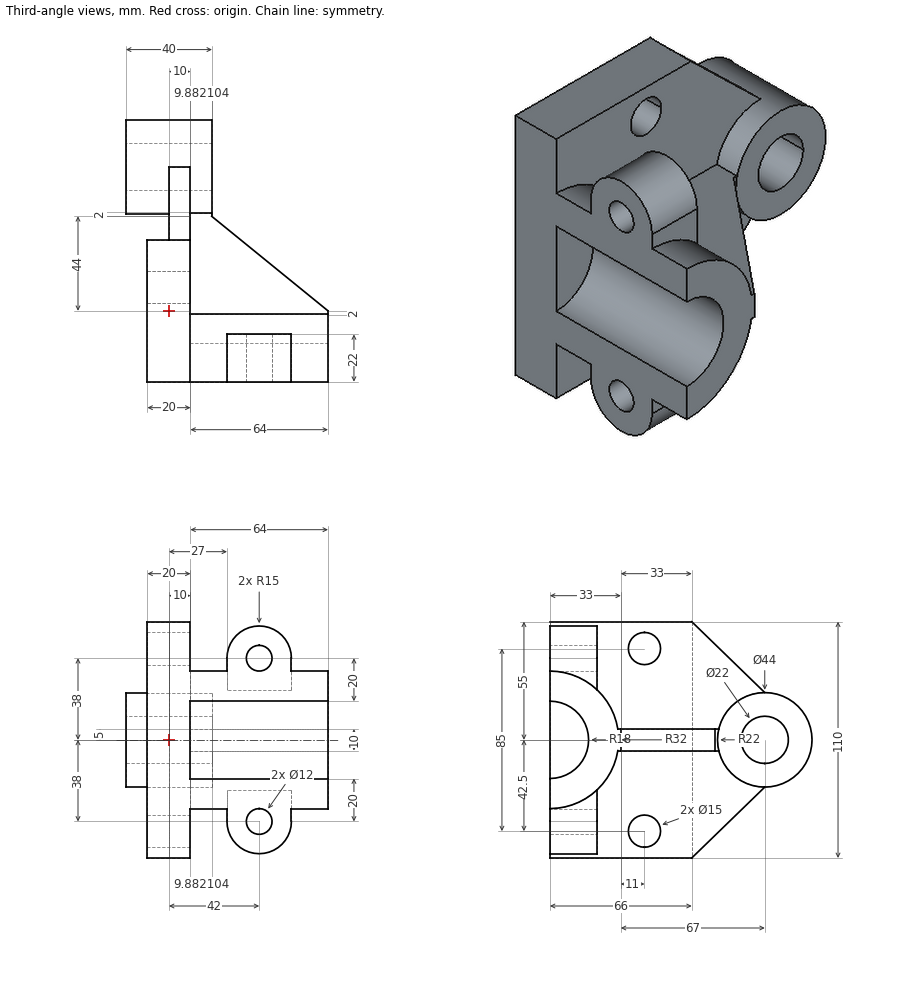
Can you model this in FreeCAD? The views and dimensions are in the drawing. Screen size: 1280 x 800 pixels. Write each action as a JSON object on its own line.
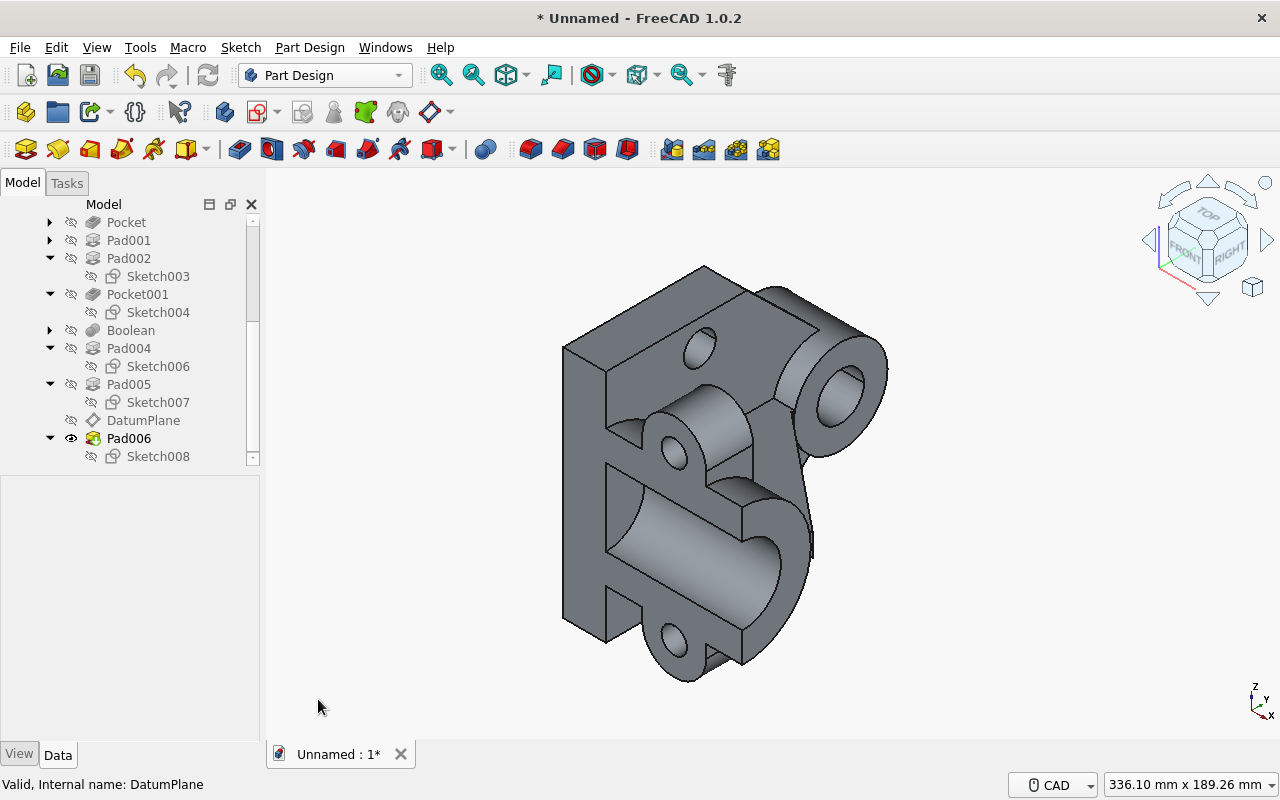
{"action": "left_click", "coordinate": [258, 112]}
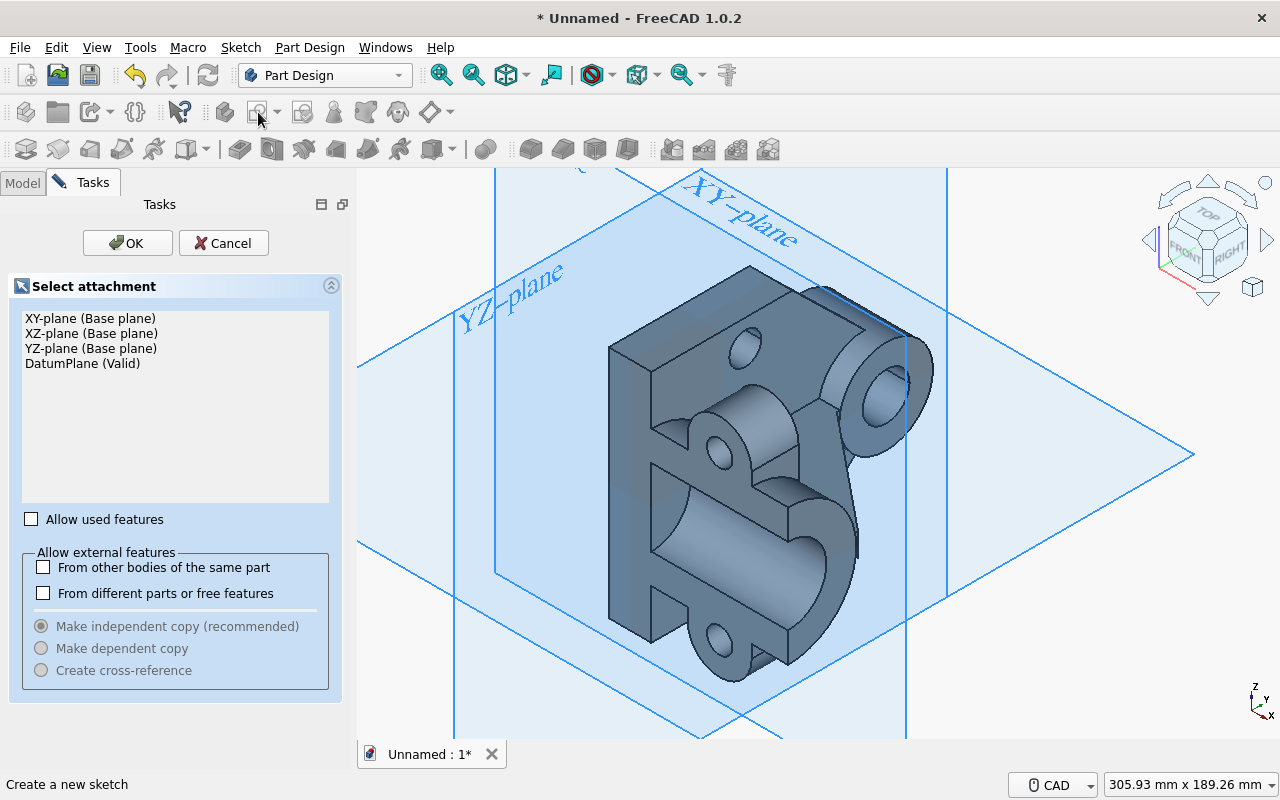
{"action": "left_click", "coordinate": [82, 334]}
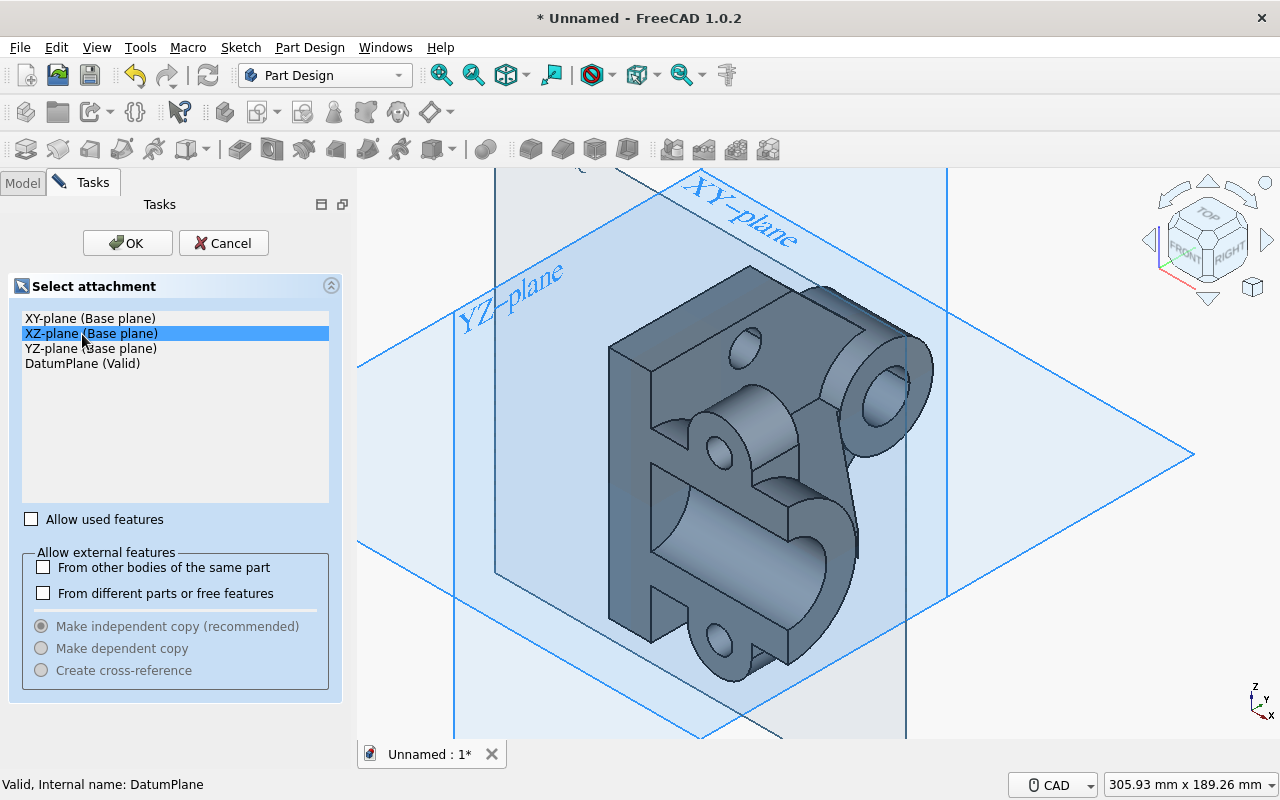
{"action": "left_click", "coordinate": [128, 243]}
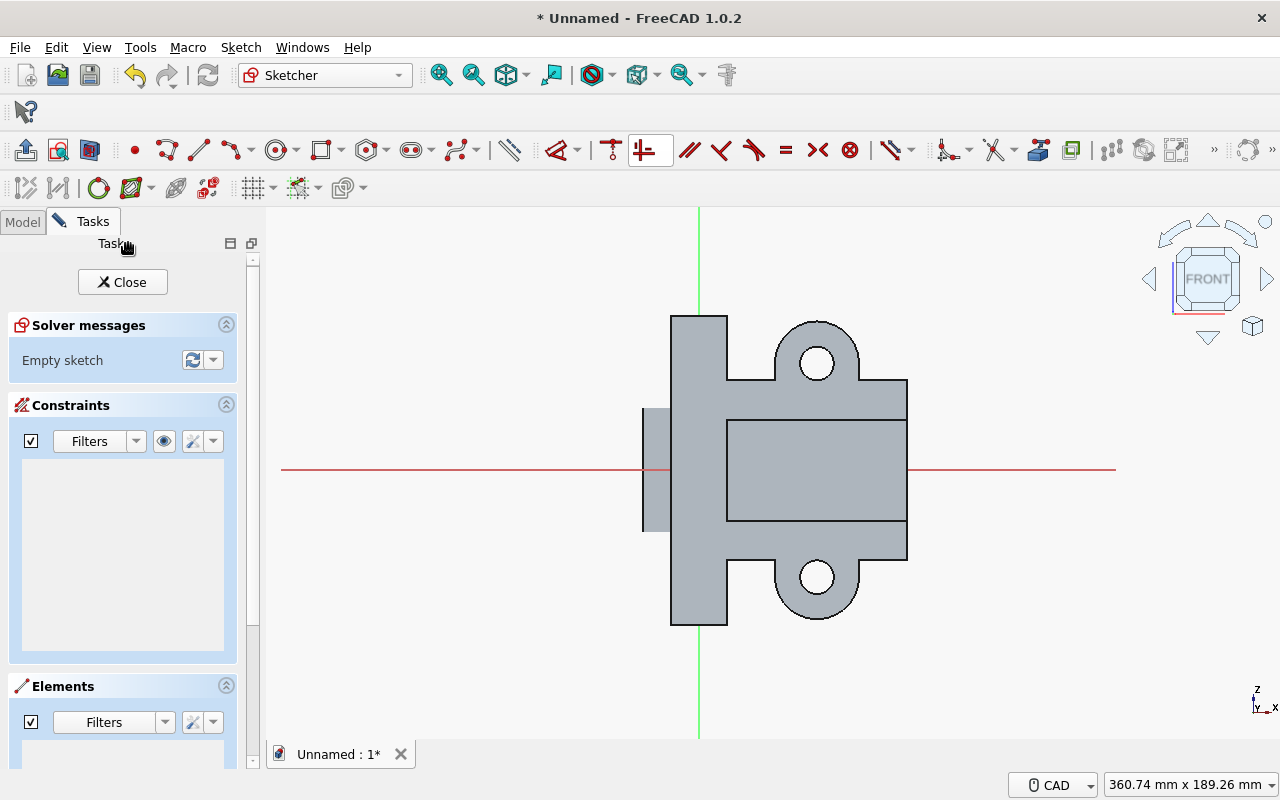
{"action": "left_click", "coordinate": [90, 150]}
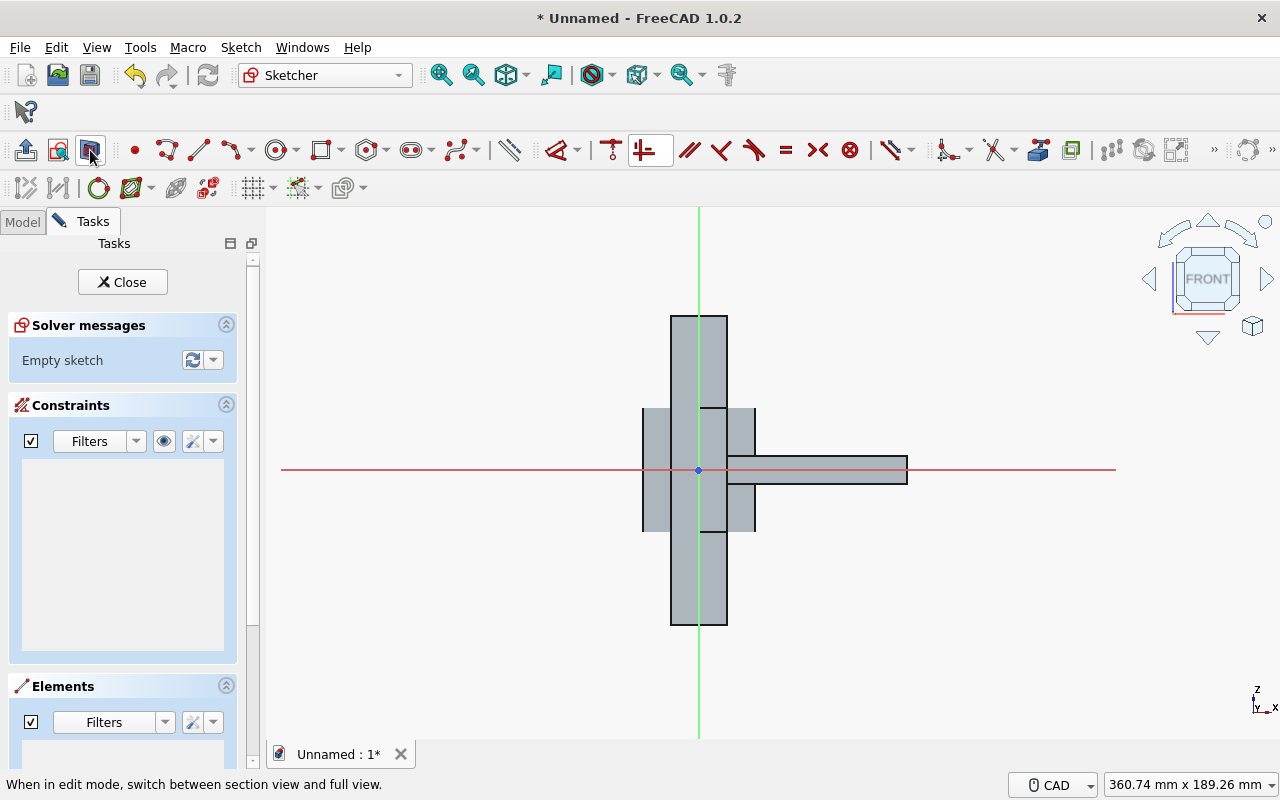
{"action": "scroll", "coordinate": [860, 469], "scroll_direction": "up", "scroll_amount": 5}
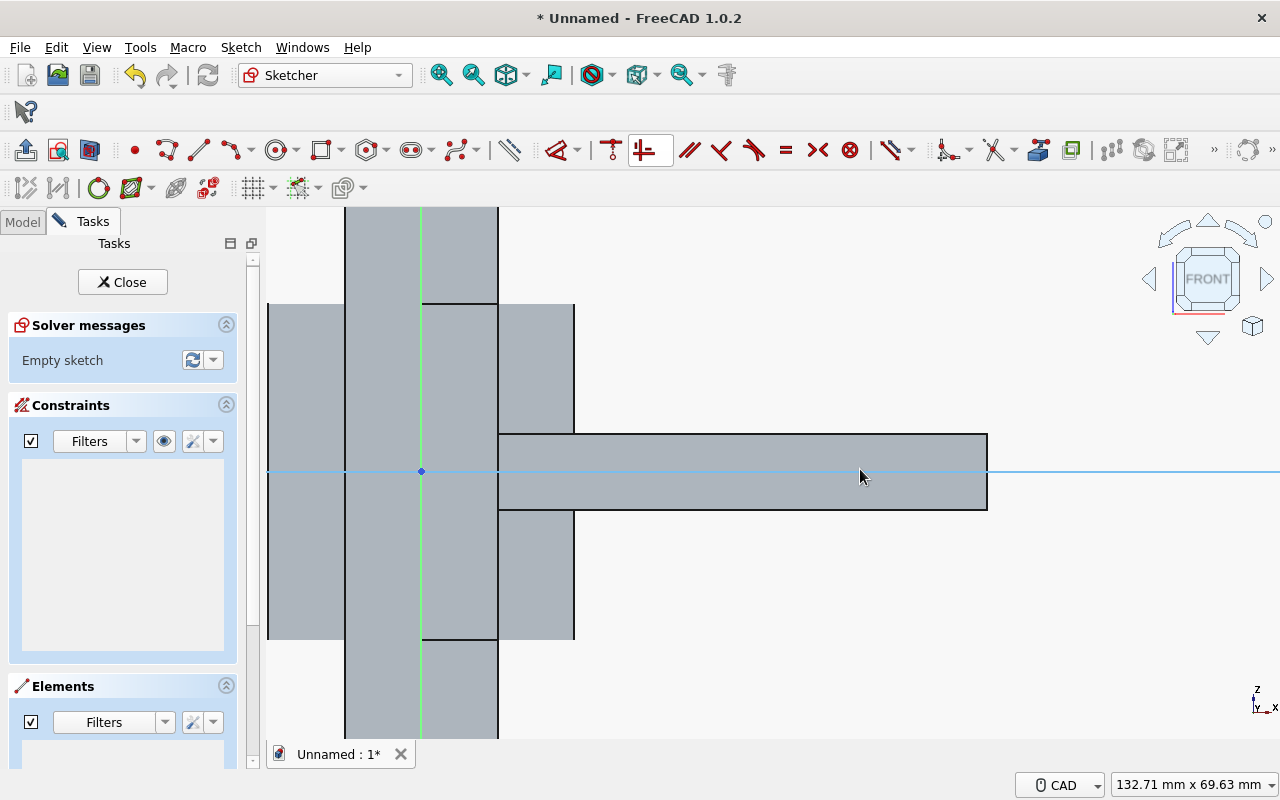
{"action": "key", "text": "g r"}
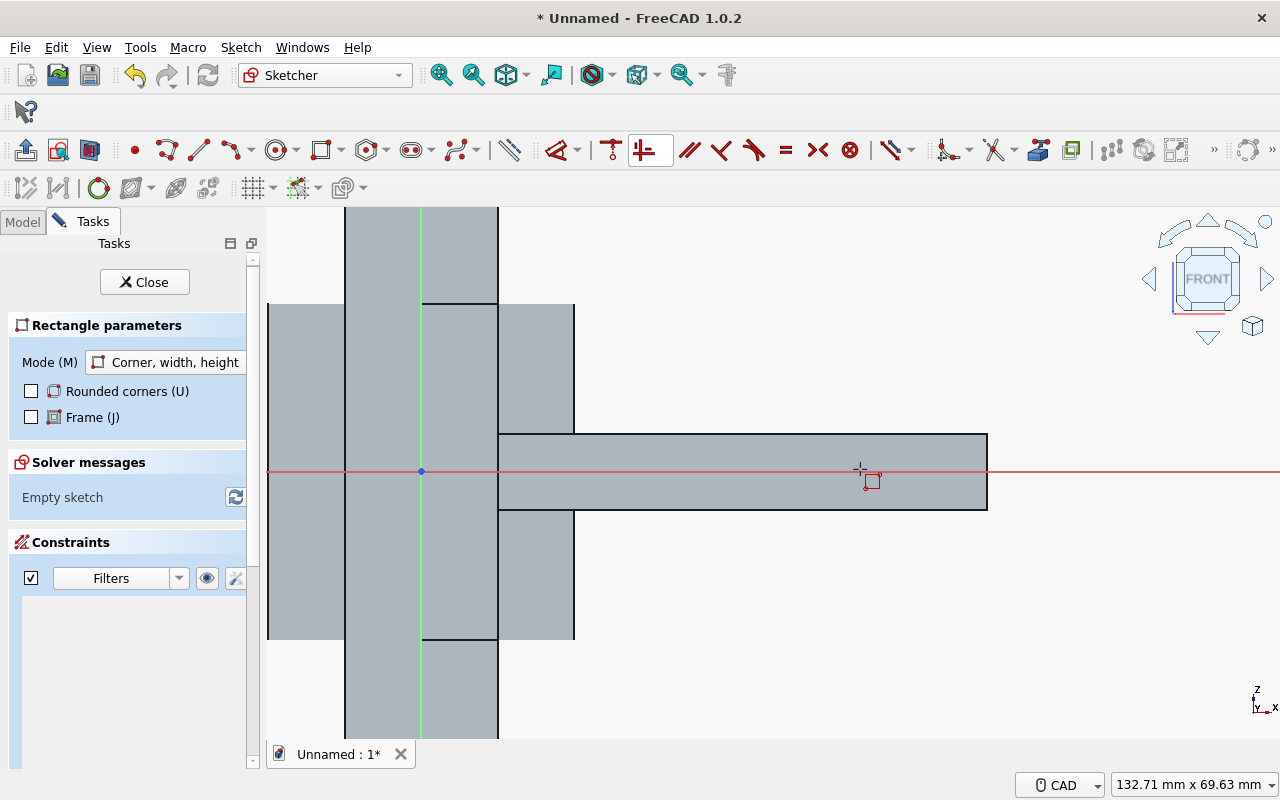
{"action": "left_click", "coordinate": [498, 434]}
{"action": "left_click", "coordinate": [987, 510]}
{"action": "key", "text": "Escape"}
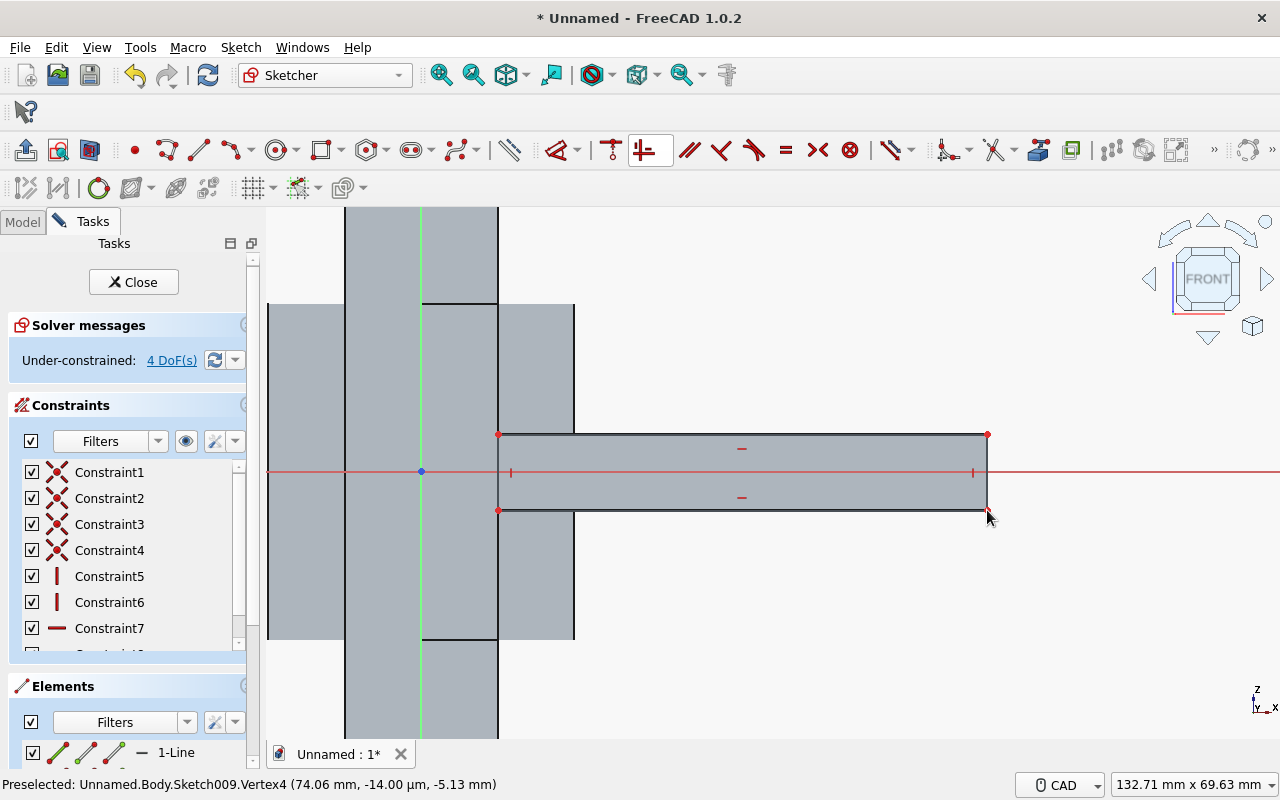
{"action": "left_click", "coordinate": [556, 150]}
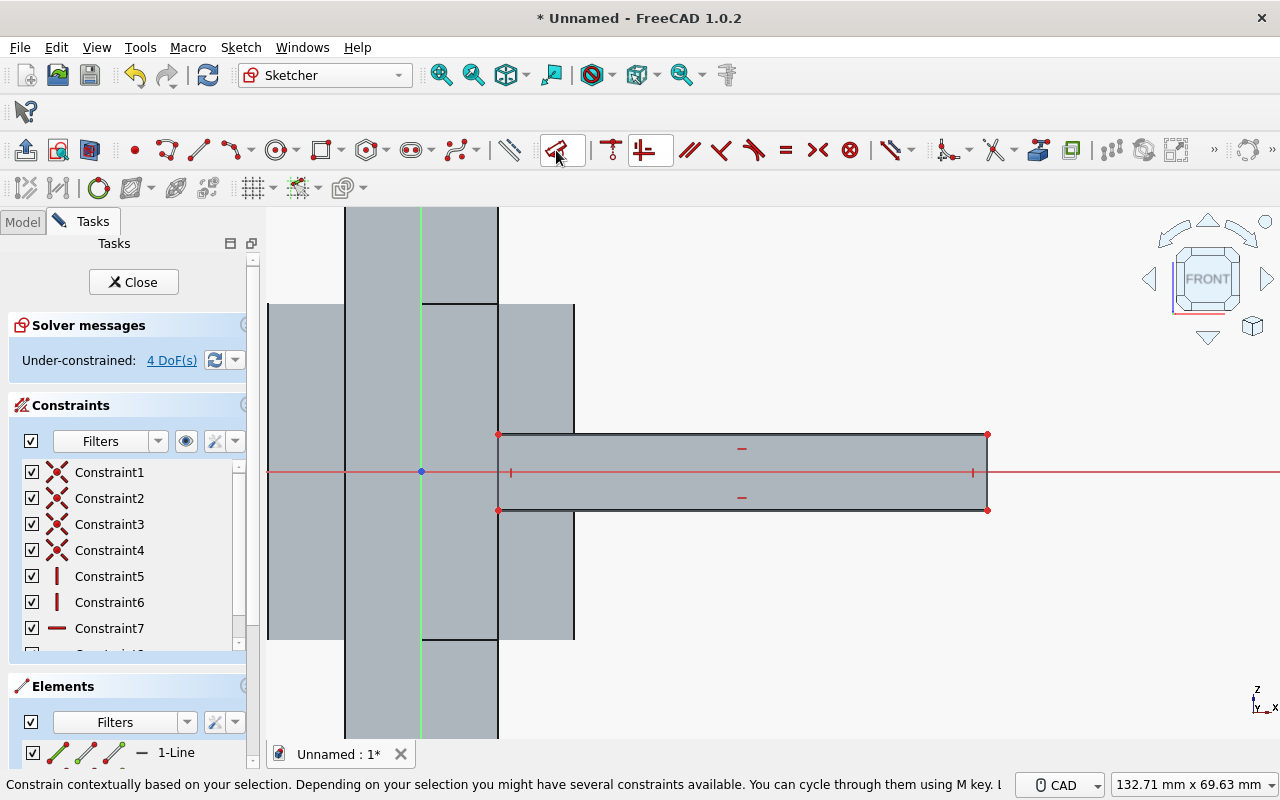
{"action": "left_click", "coordinate": [498, 458]}
{"action": "left_click", "coordinate": [464, 456]}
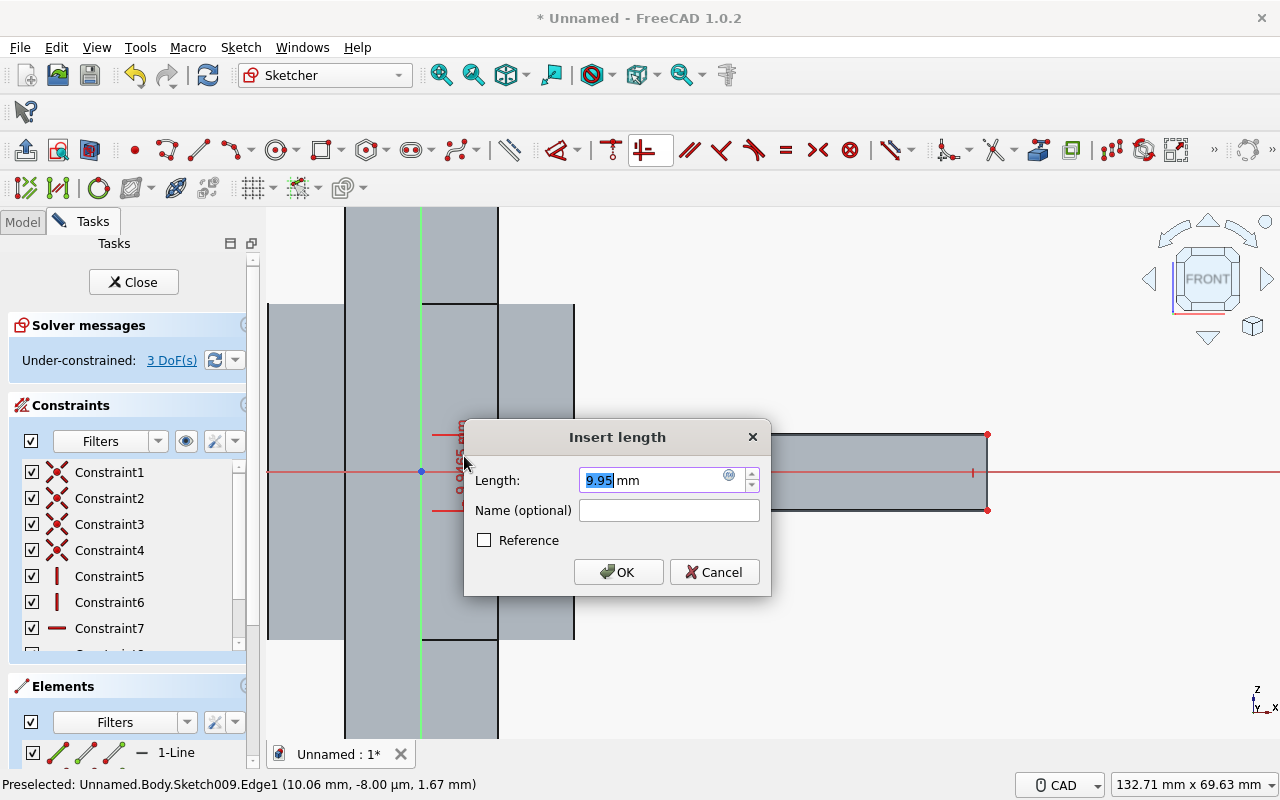
{"action": "type", "text": "10"}
{"action": "key", "text": "Return"}